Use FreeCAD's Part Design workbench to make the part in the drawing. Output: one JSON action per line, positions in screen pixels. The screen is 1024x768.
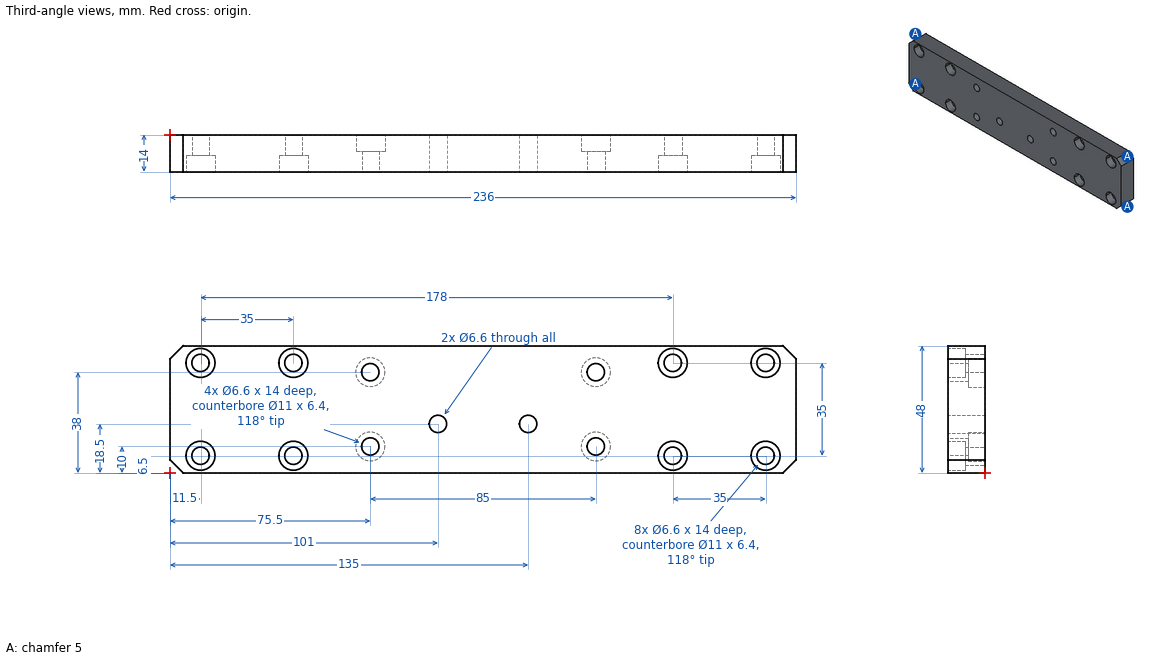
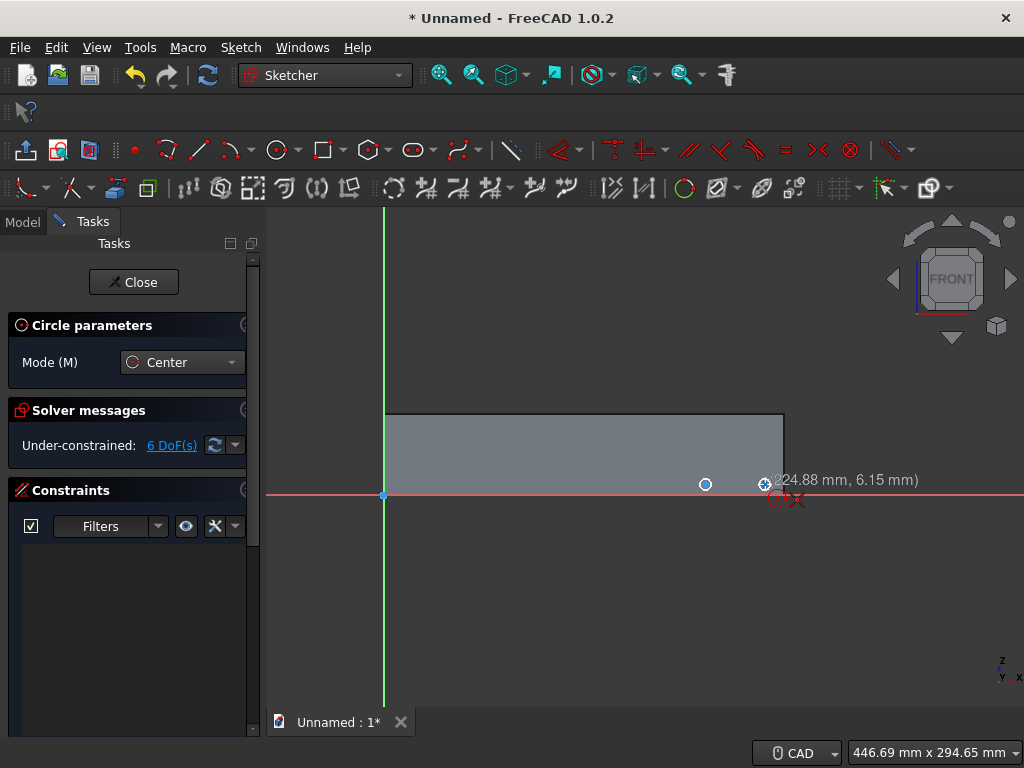
{"action": "left_click", "coordinate": [705, 425]}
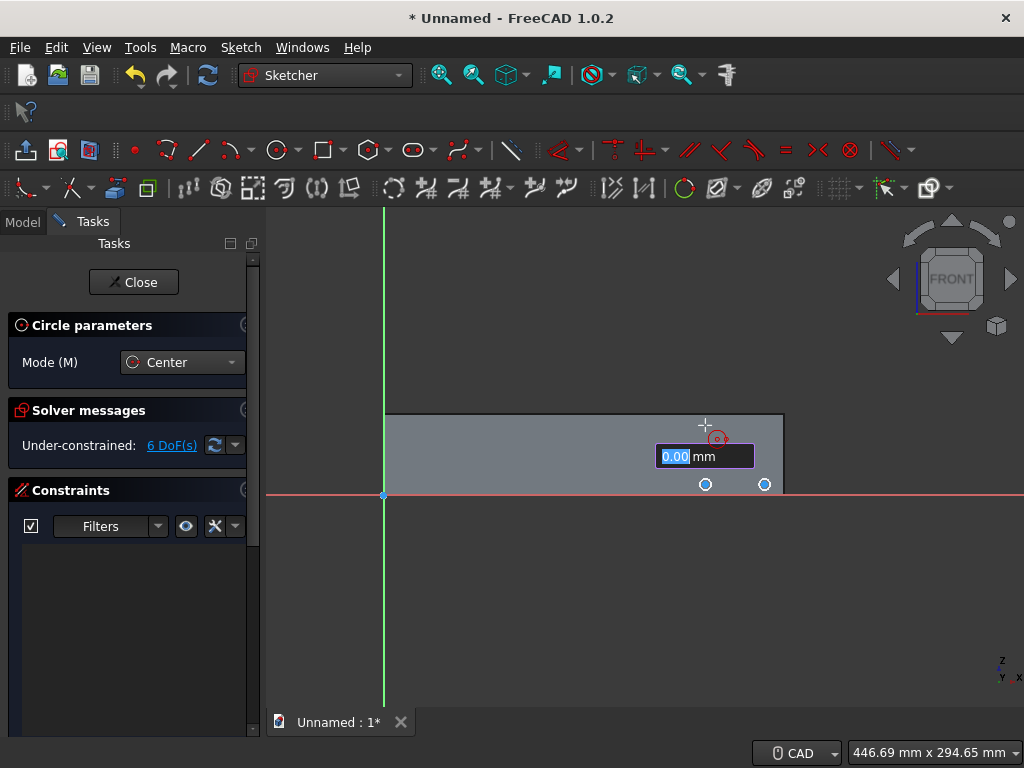
{"action": "scroll", "coordinate": [709, 421], "scroll_direction": "up", "scroll_amount": 6}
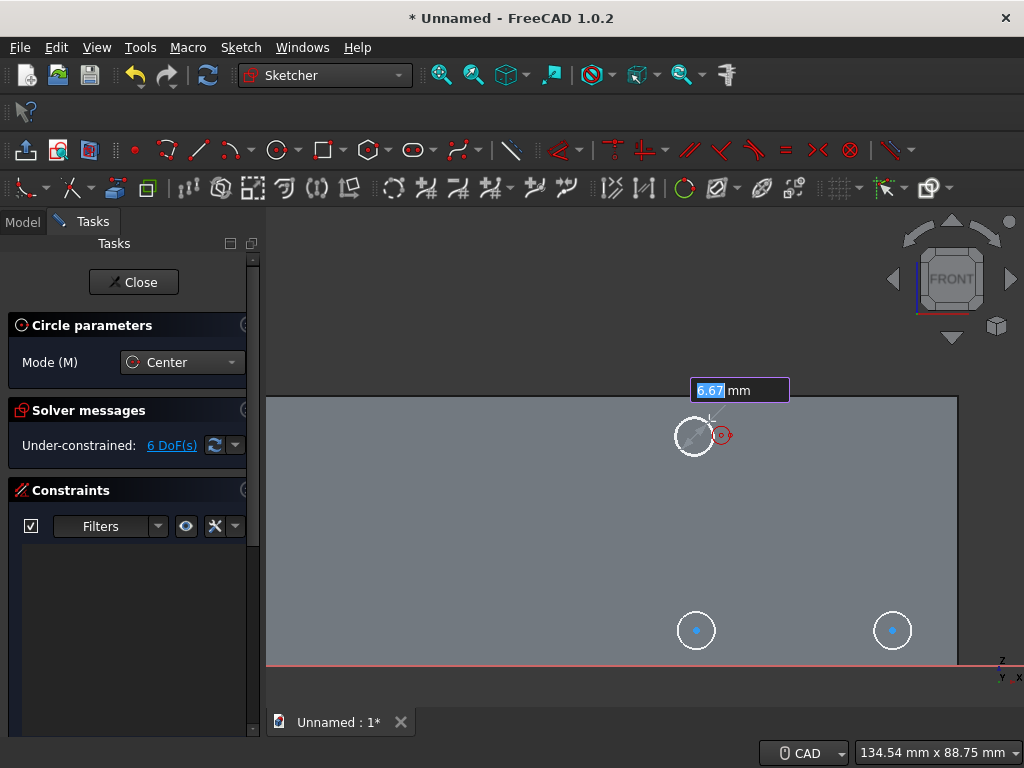
{"action": "left_click", "coordinate": [709, 419]}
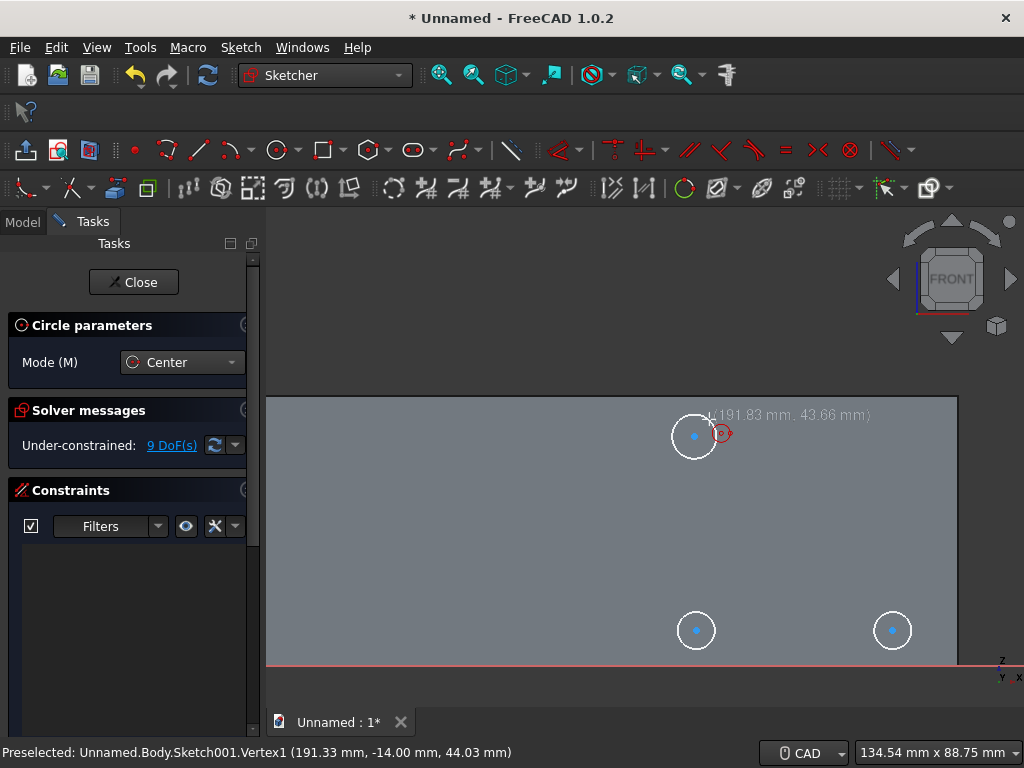
{"action": "scroll", "coordinate": [709, 421], "scroll_direction": "down", "scroll_amount": 6}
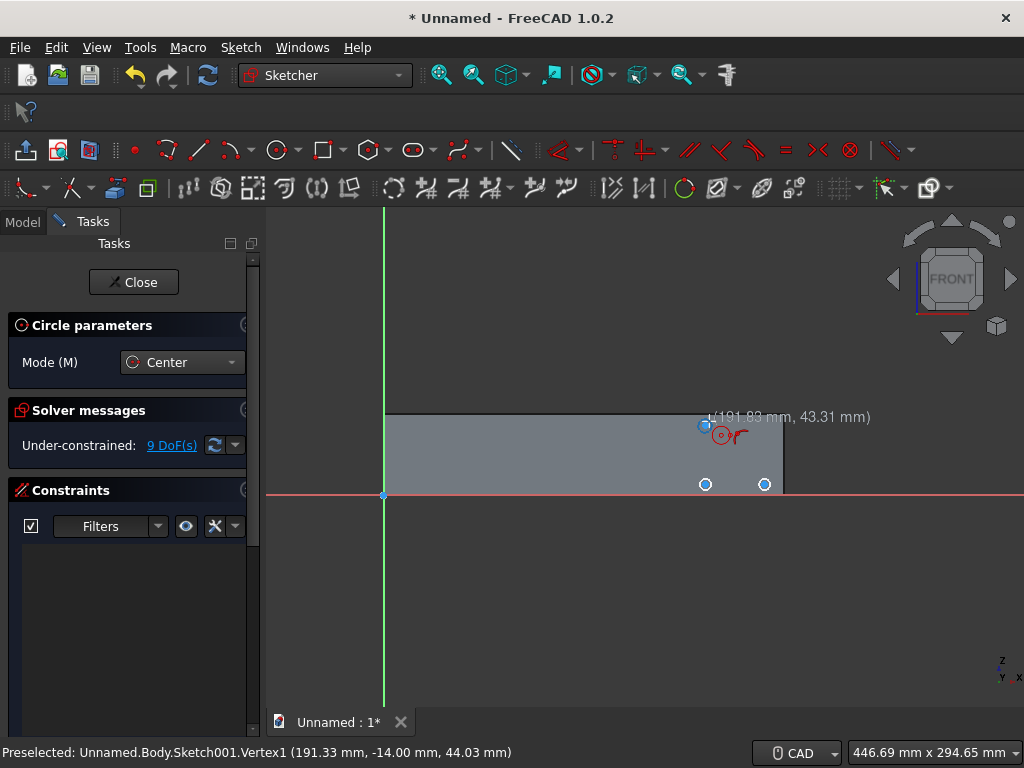
{"action": "scroll", "coordinate": [765, 425], "scroll_direction": "up", "scroll_amount": 7}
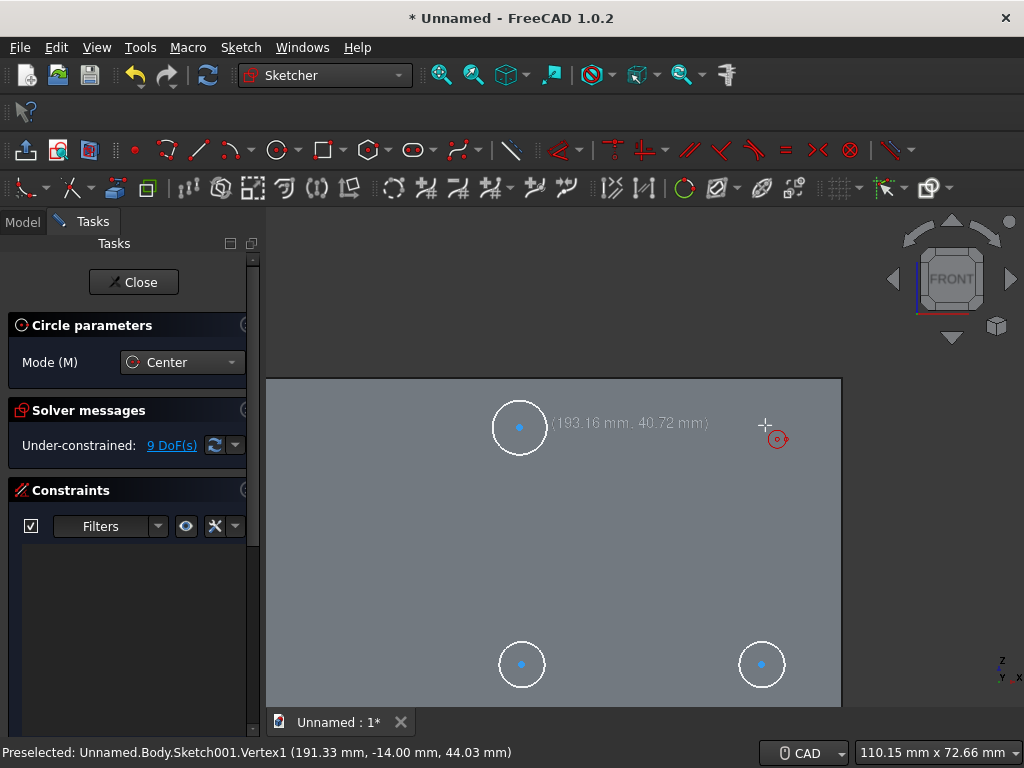
{"action": "scroll", "coordinate": [765, 425], "scroll_direction": "down", "scroll_amount": 7}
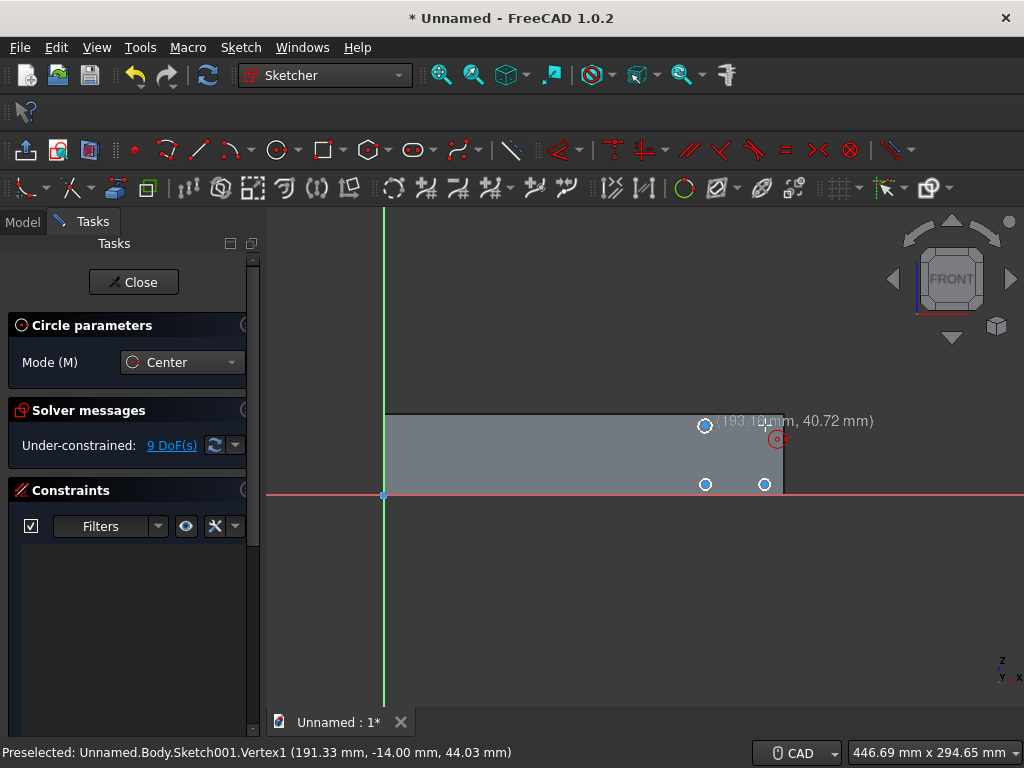
{"action": "left_click", "coordinate": [765, 425]}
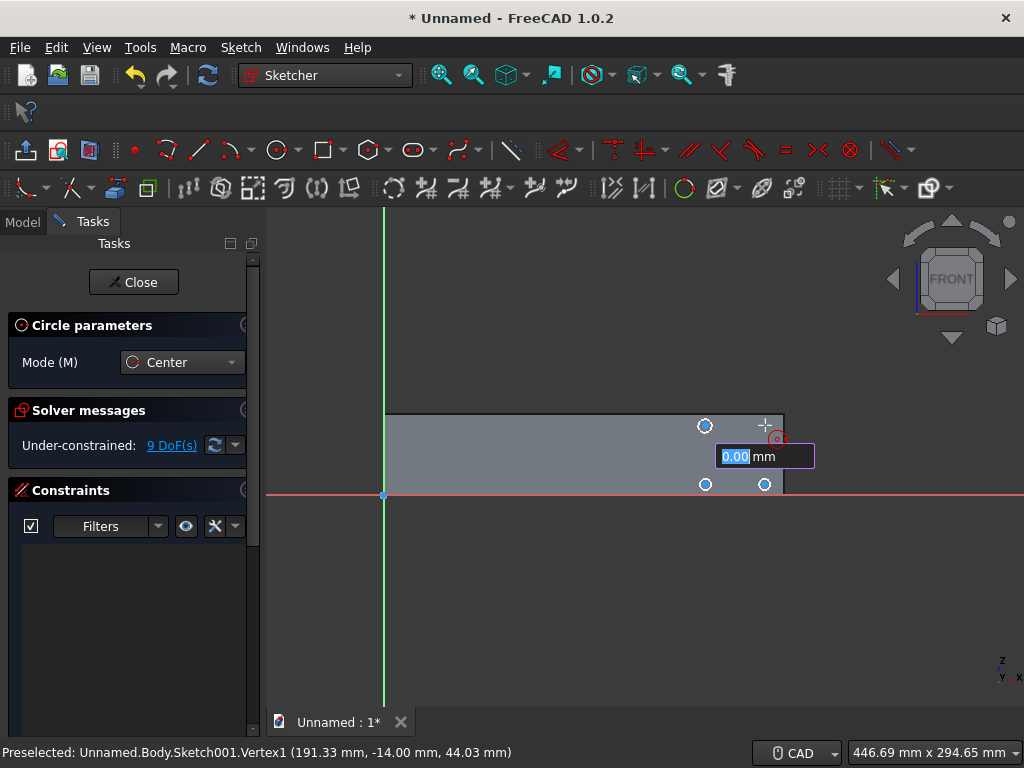
{"action": "scroll", "coordinate": [769, 421], "scroll_direction": "up", "scroll_amount": 6}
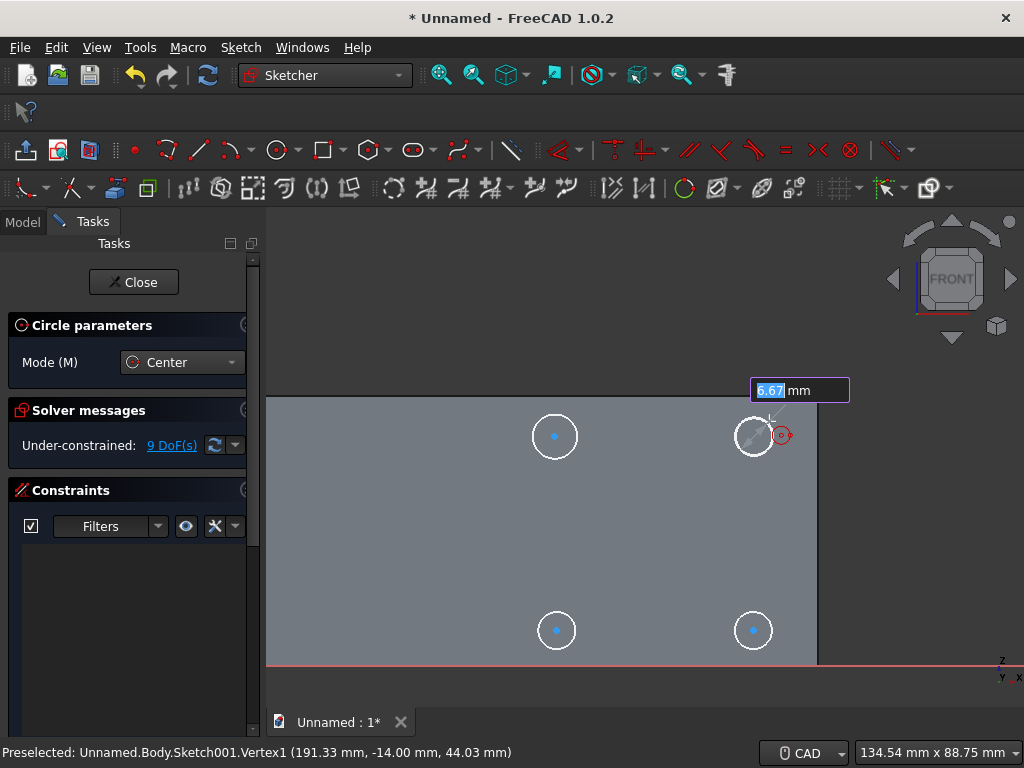
{"action": "left_click", "coordinate": [767, 419]}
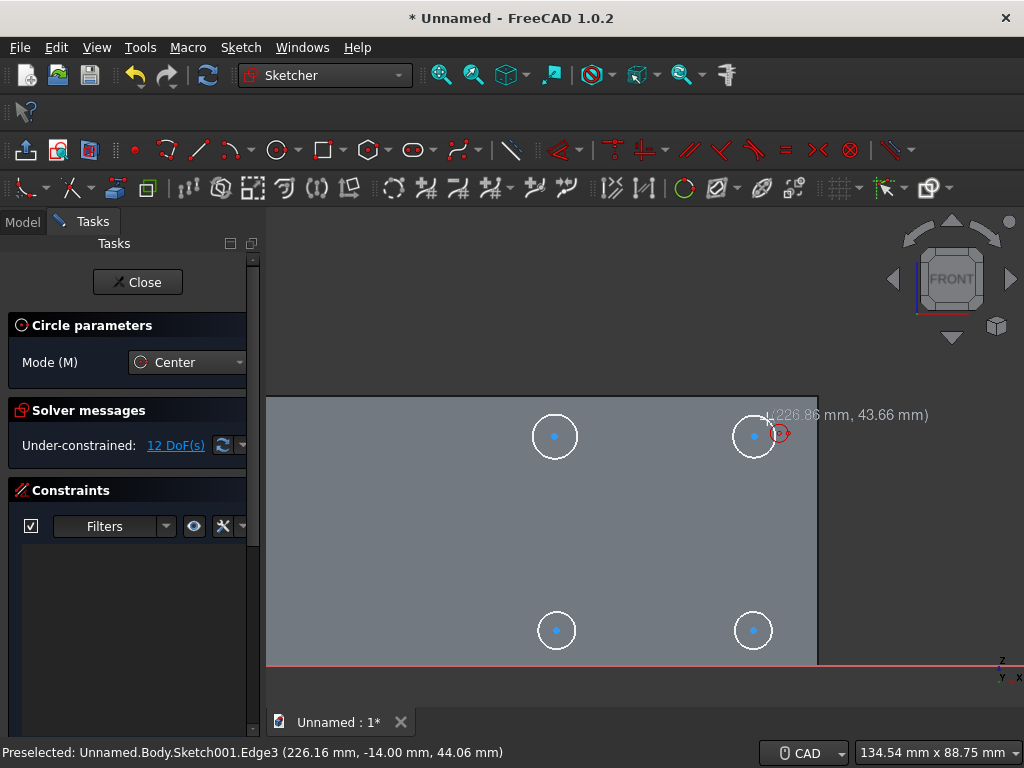
{"action": "scroll", "coordinate": [769, 421], "scroll_direction": "down", "scroll_amount": 6}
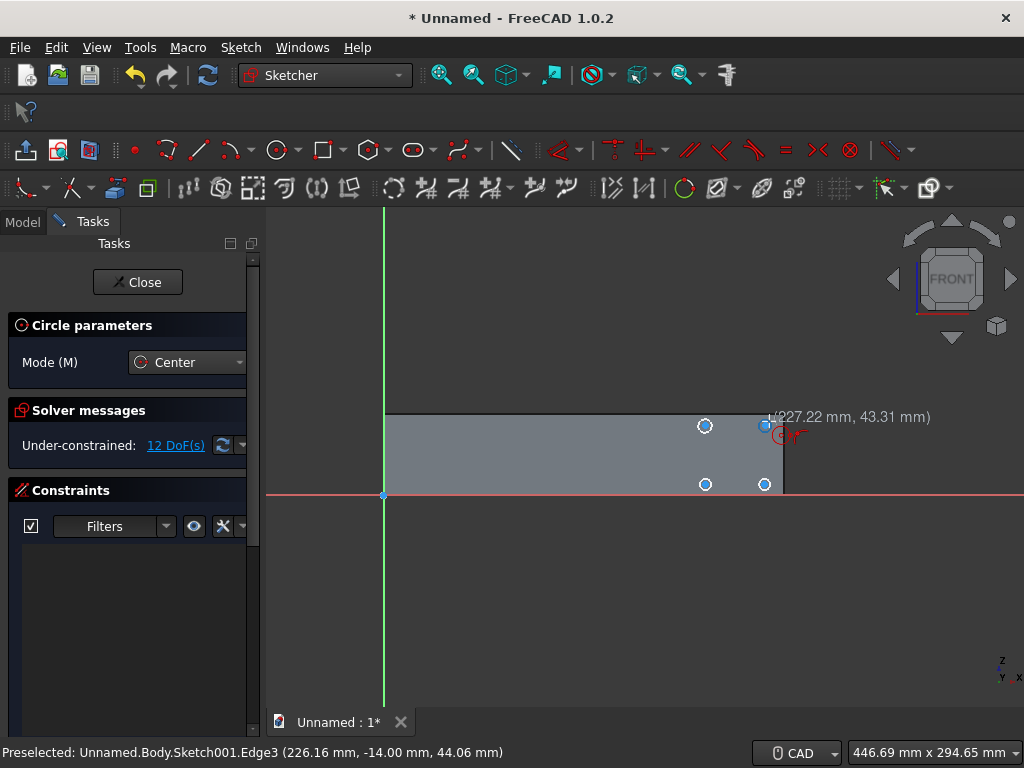
{"action": "scroll", "coordinate": [403, 425], "scroll_direction": "up", "scroll_amount": 7}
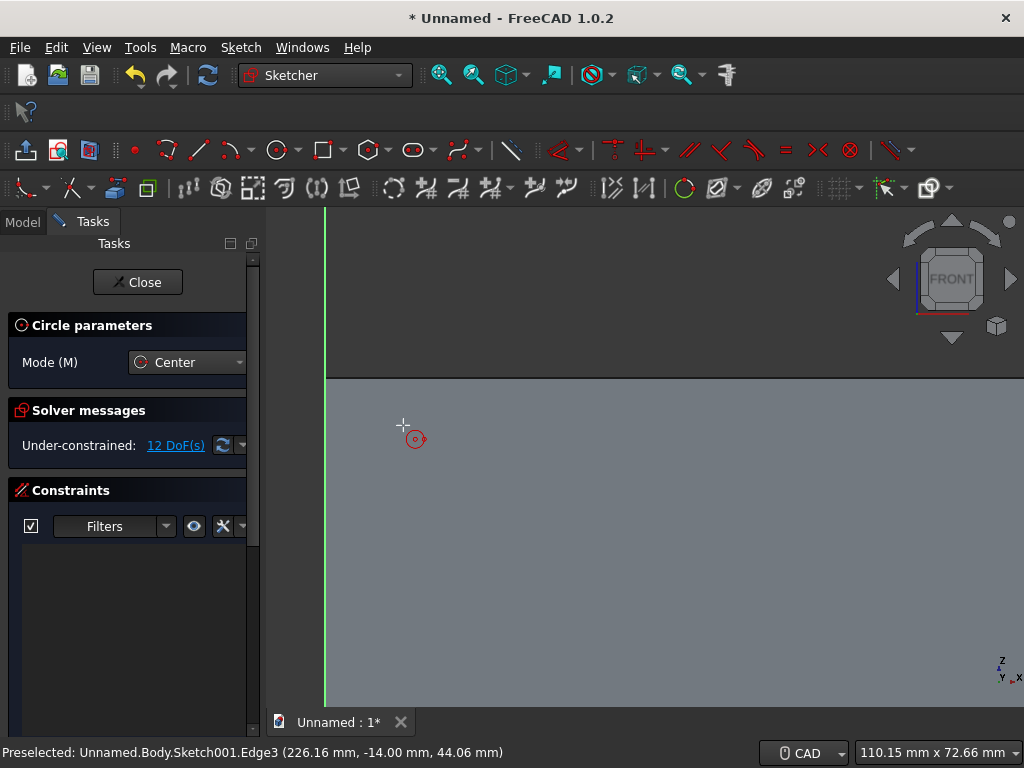
{"action": "scroll", "coordinate": [402, 425], "scroll_direction": "down", "scroll_amount": 7}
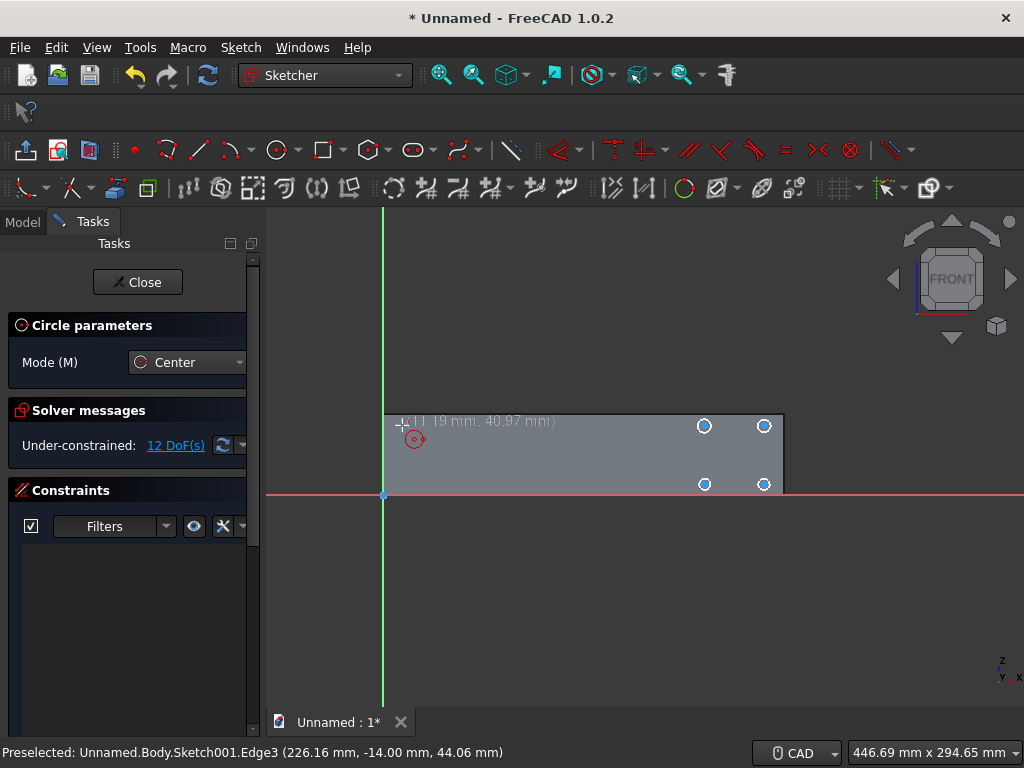
{"action": "left_click", "coordinate": [403, 425]}